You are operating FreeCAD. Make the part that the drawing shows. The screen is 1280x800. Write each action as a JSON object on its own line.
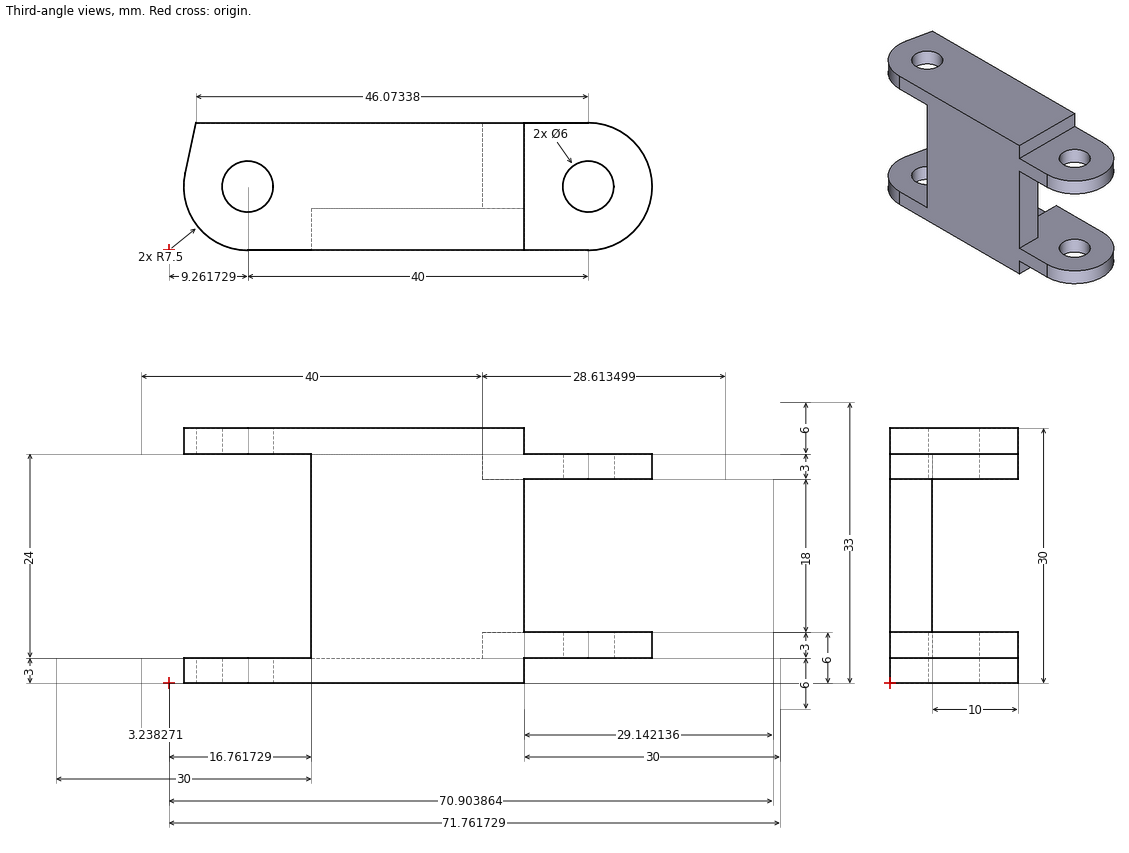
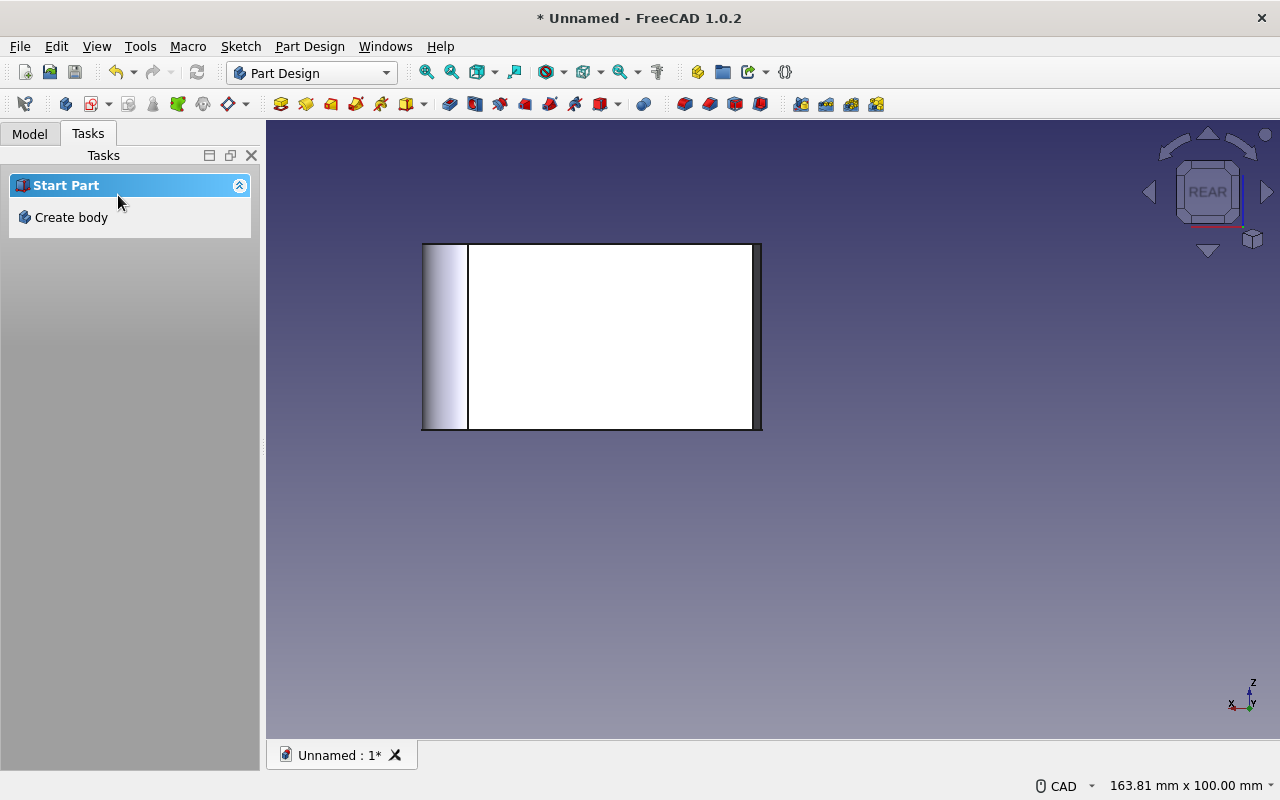
{"action": "left_click", "coordinate": [427, 72]}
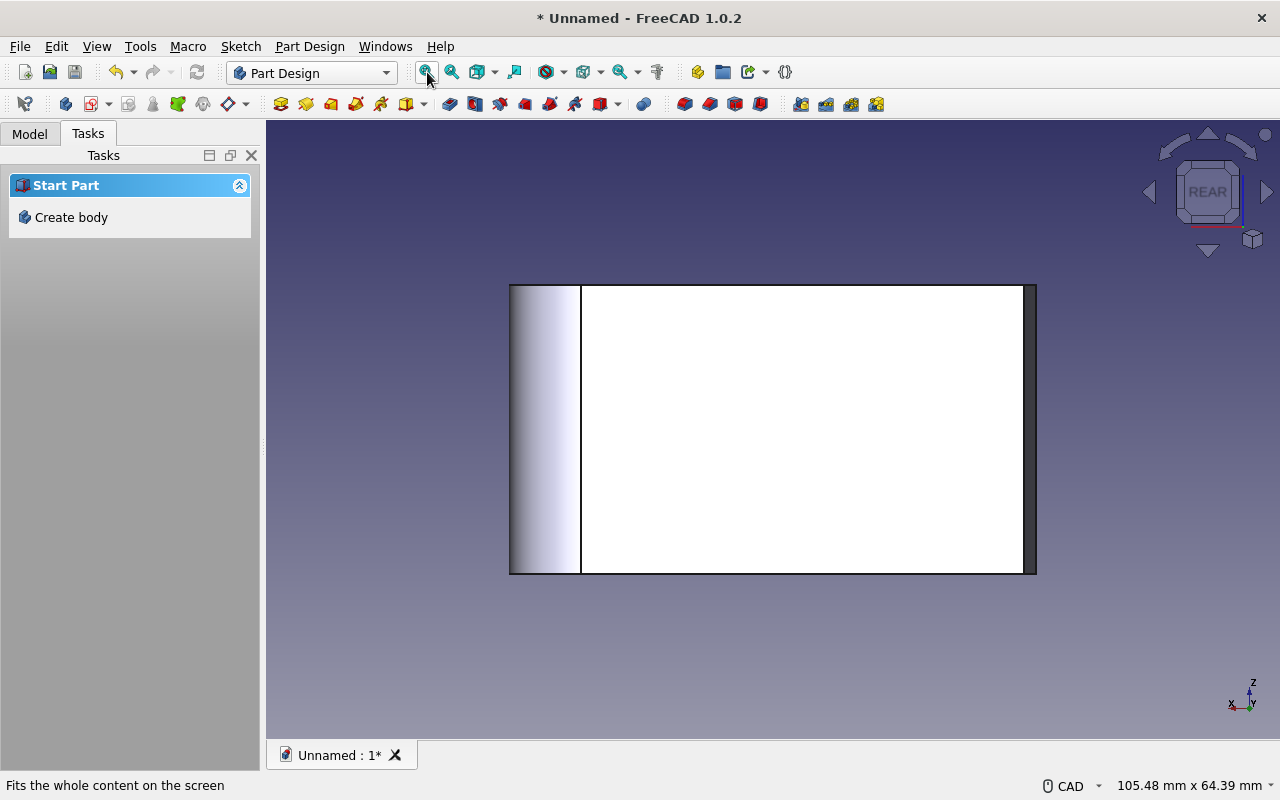
{"action": "left_click", "coordinate": [739, 429]}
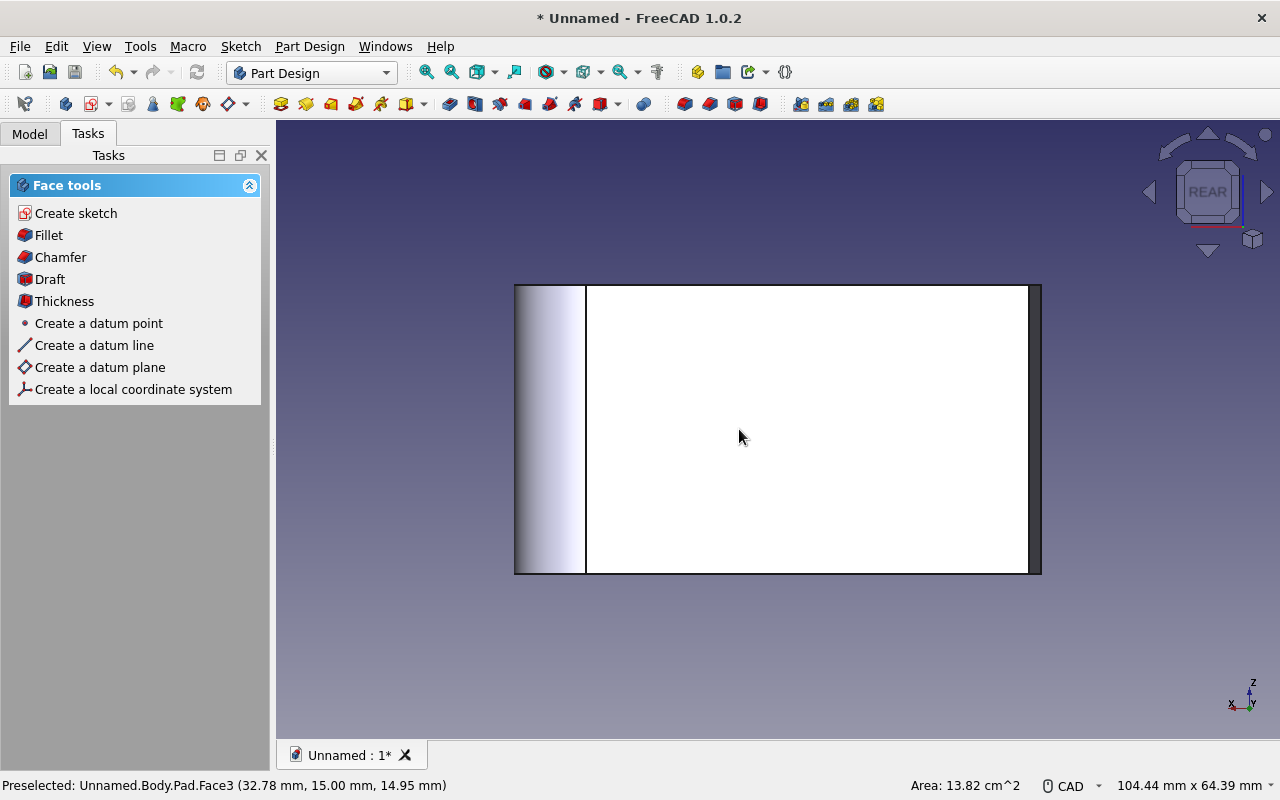
{"action": "left_click", "coordinate": [90, 104]}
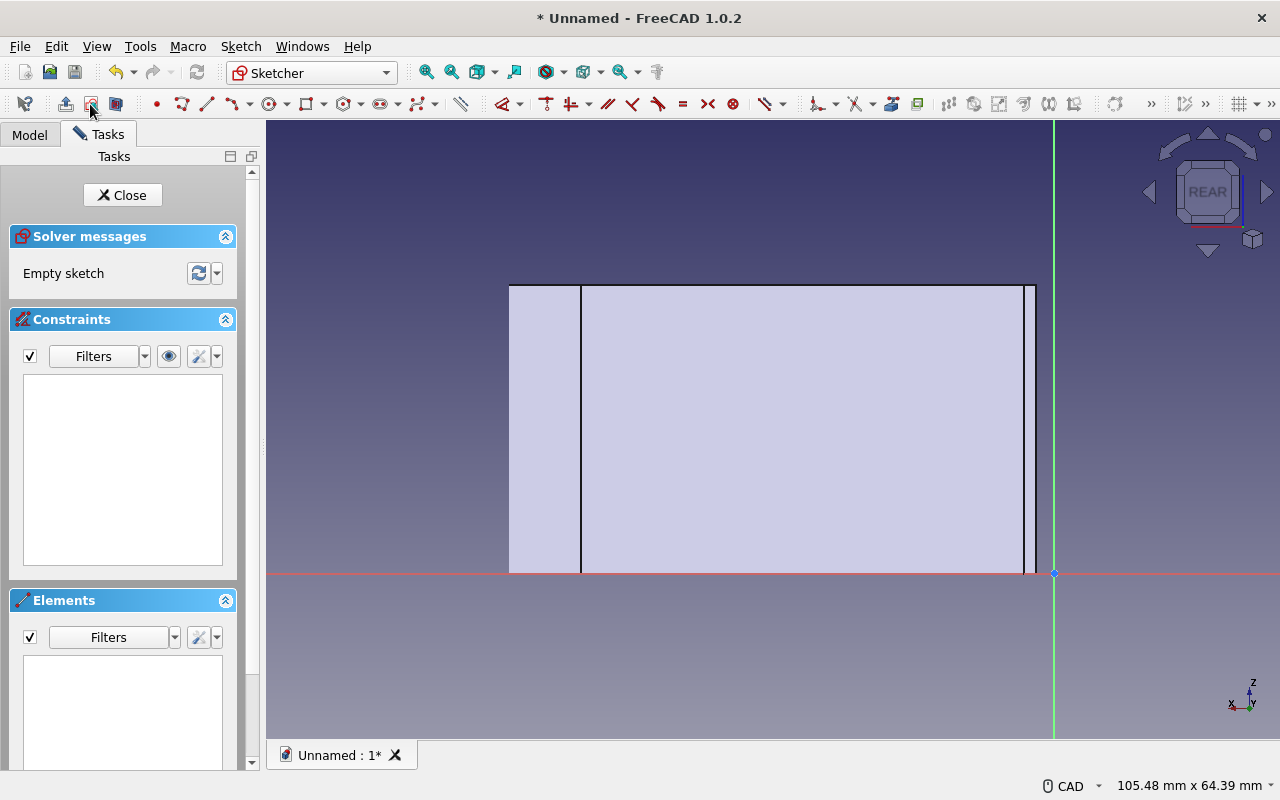
{"action": "scroll", "coordinate": [565, 429], "scroll_direction": "down", "scroll_amount": 2}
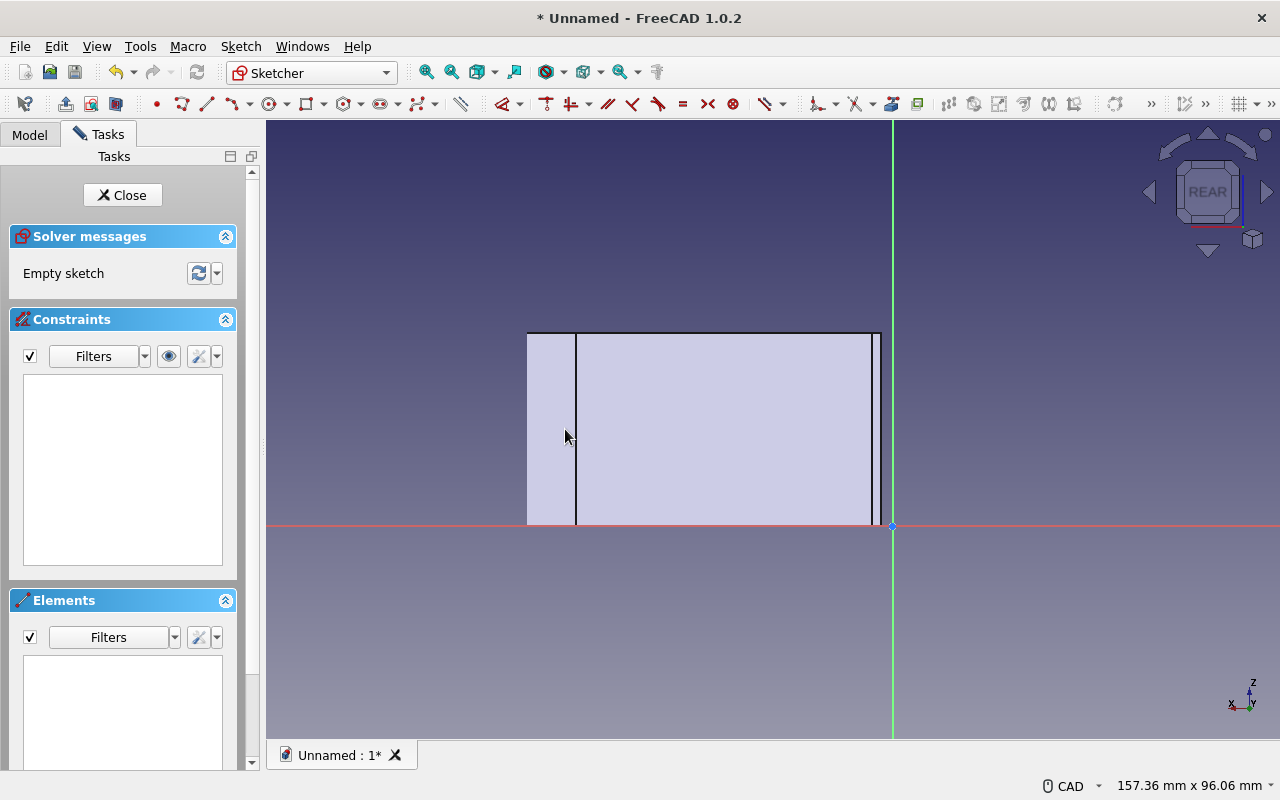
{"action": "left_click", "coordinate": [306, 104]}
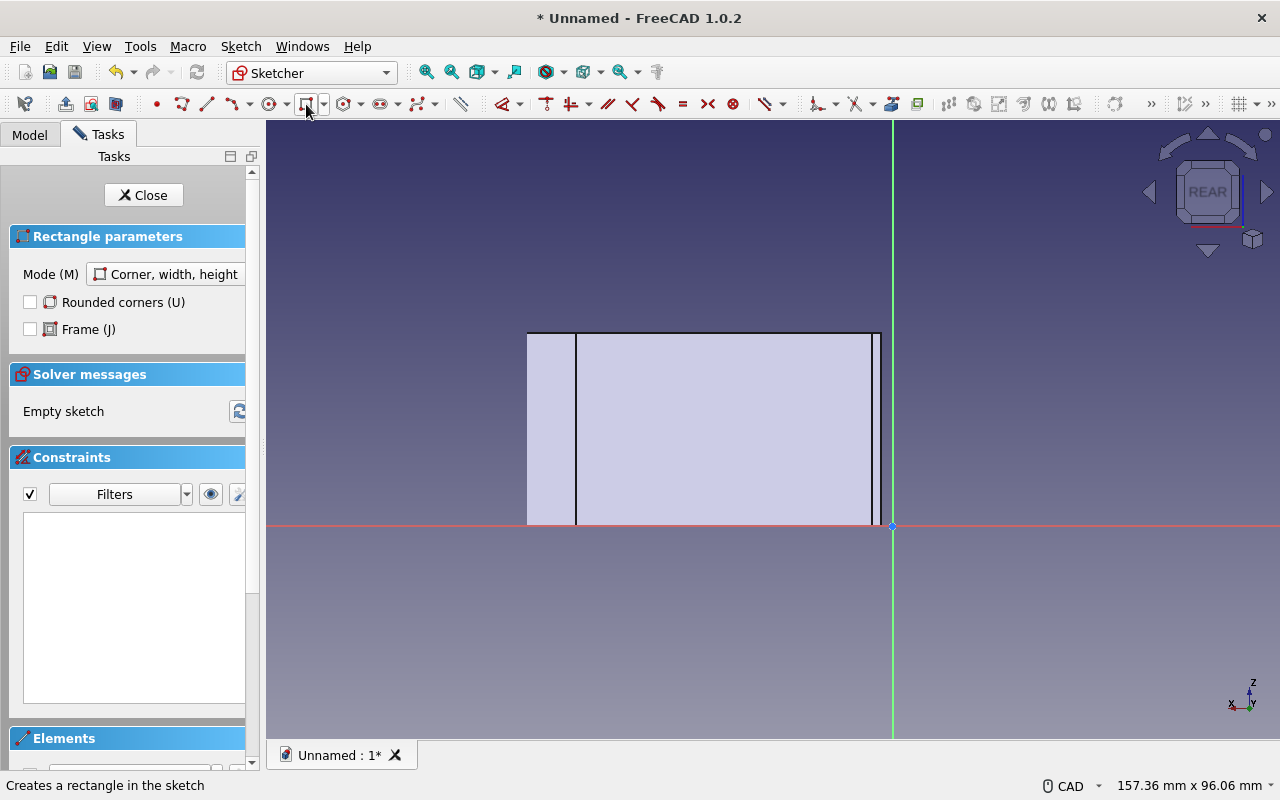
{"action": "left_click", "coordinate": [785, 352]}
{"action": "left_click", "coordinate": [978, 507]}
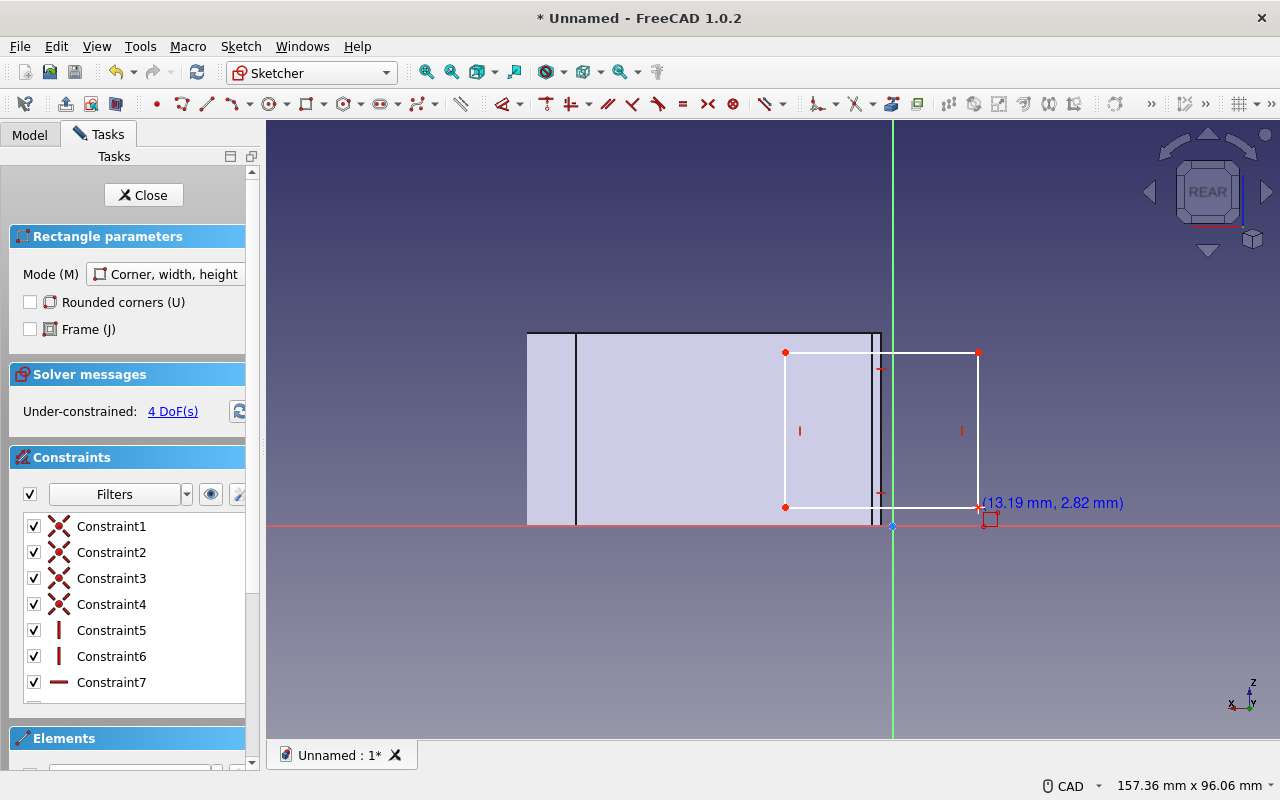
{"action": "left_click", "coordinate": [431, 507]}
{"action": "left_click", "coordinate": [624, 545]}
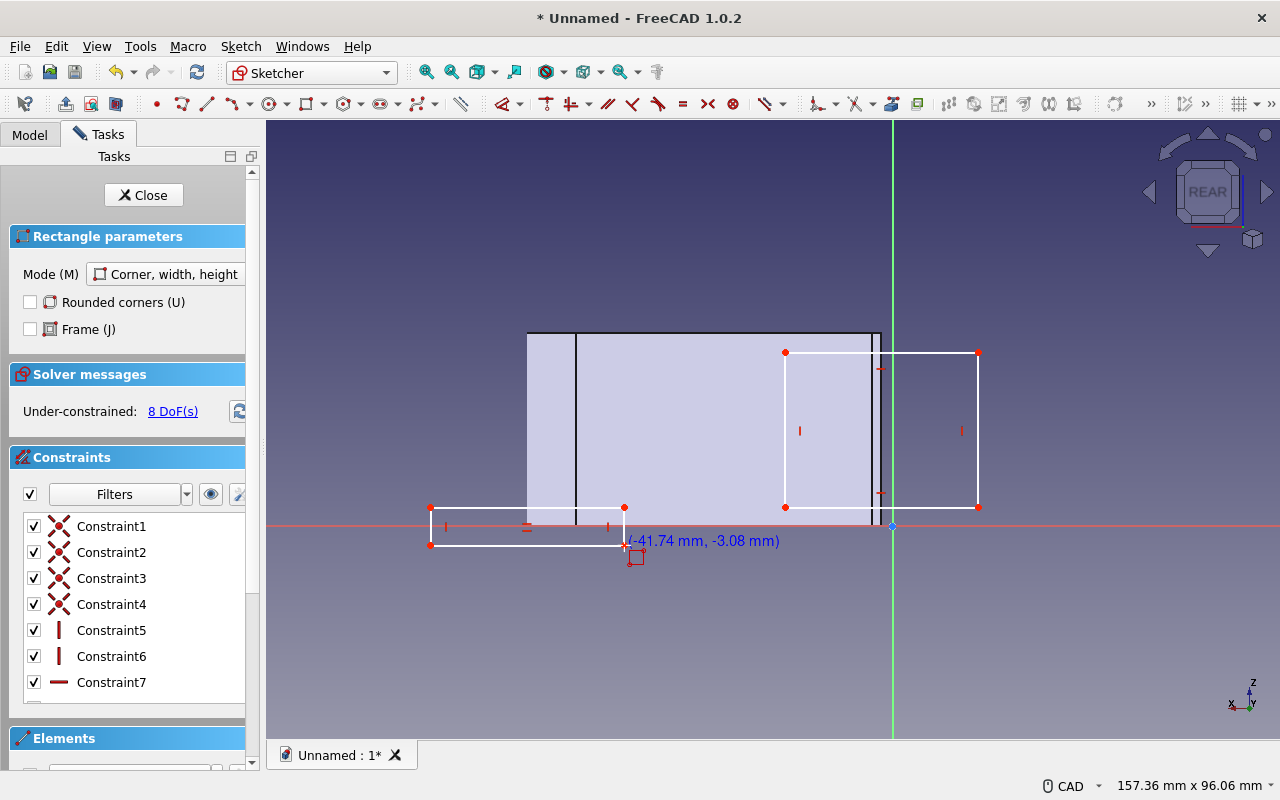
{"action": "left_click", "coordinate": [431, 314]}
{"action": "left_click", "coordinate": [624, 352]}
{"action": "key", "text": "Escape"}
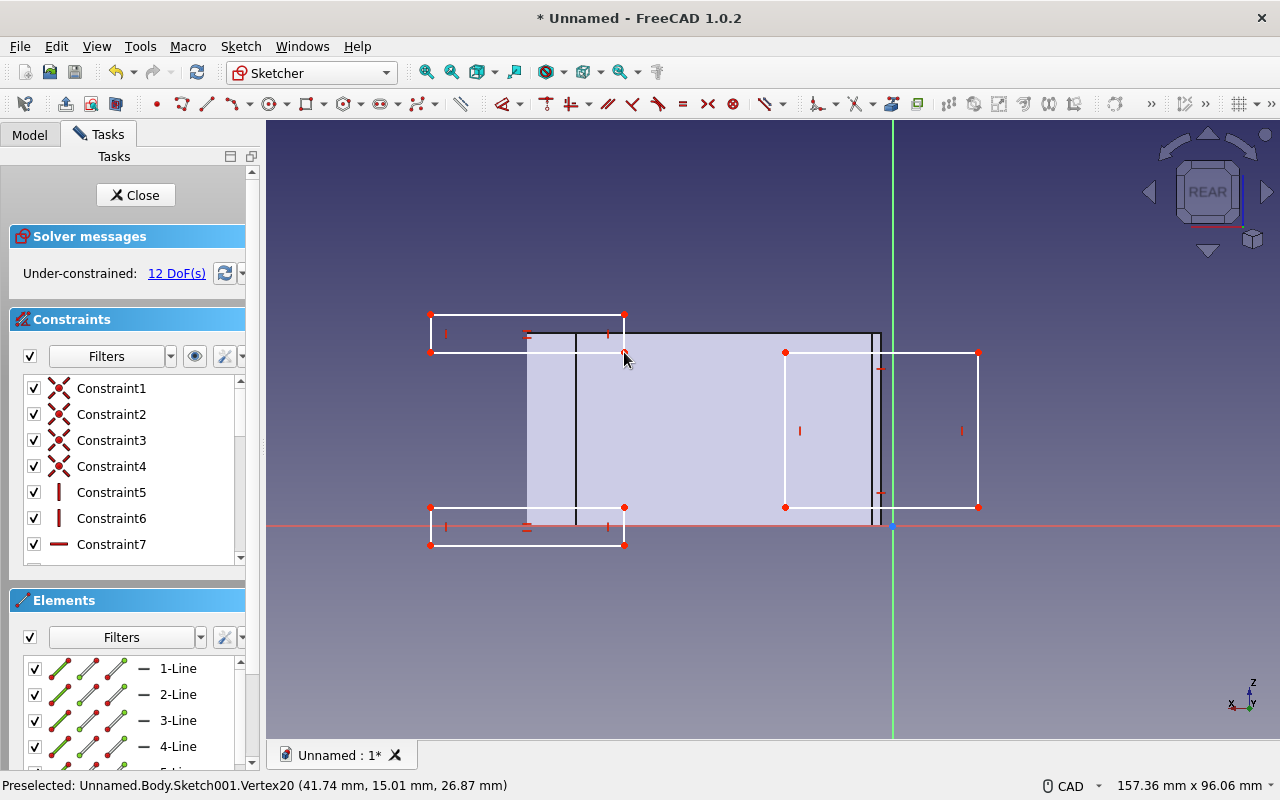
{"action": "left_click", "coordinate": [502, 104]}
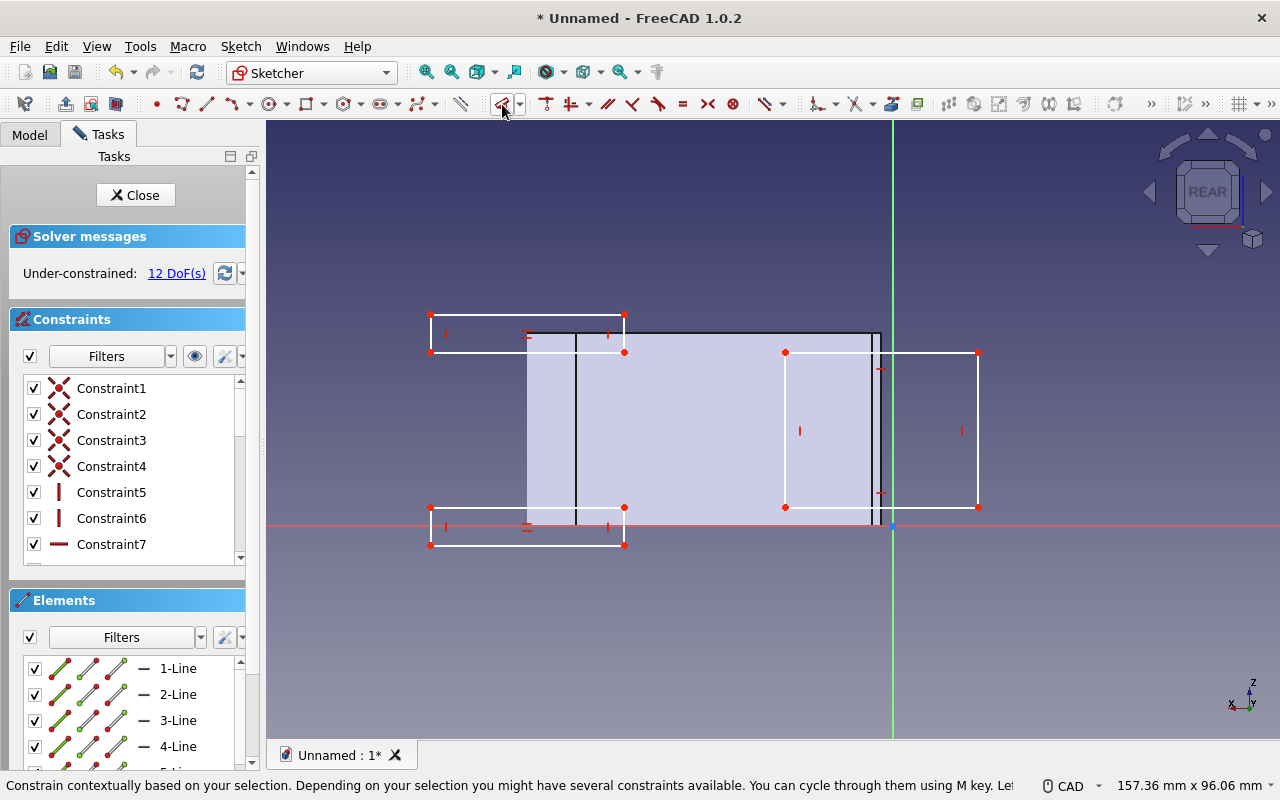
{"action": "left_click", "coordinate": [431, 523]}
{"action": "left_click", "coordinate": [397, 540]}